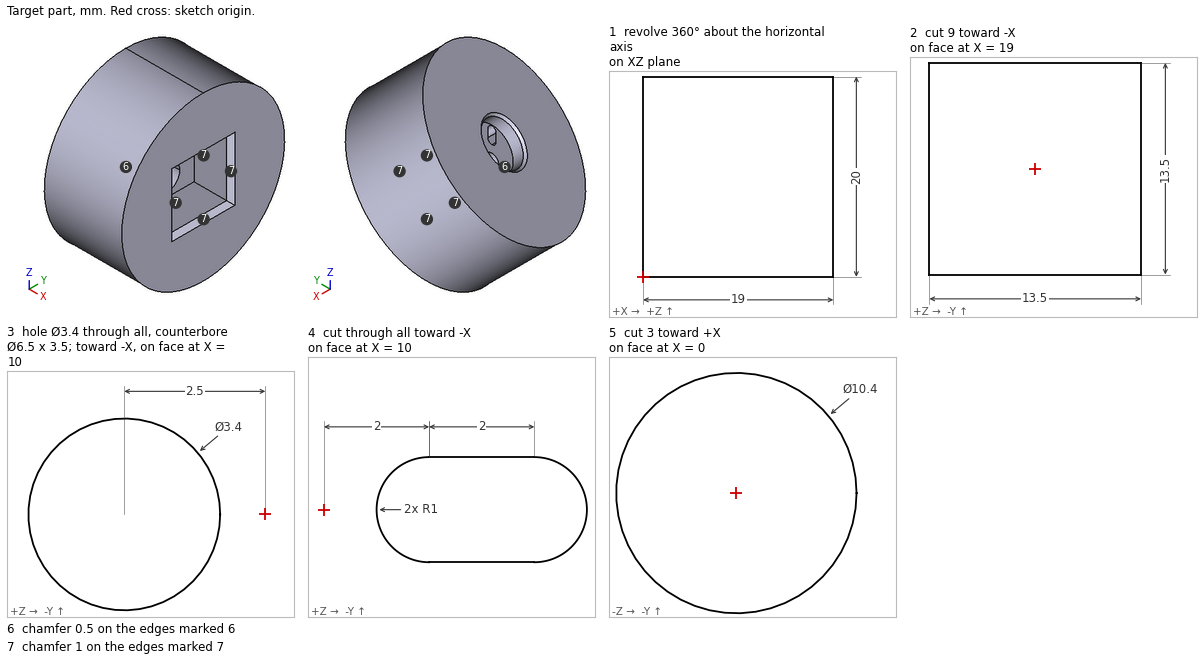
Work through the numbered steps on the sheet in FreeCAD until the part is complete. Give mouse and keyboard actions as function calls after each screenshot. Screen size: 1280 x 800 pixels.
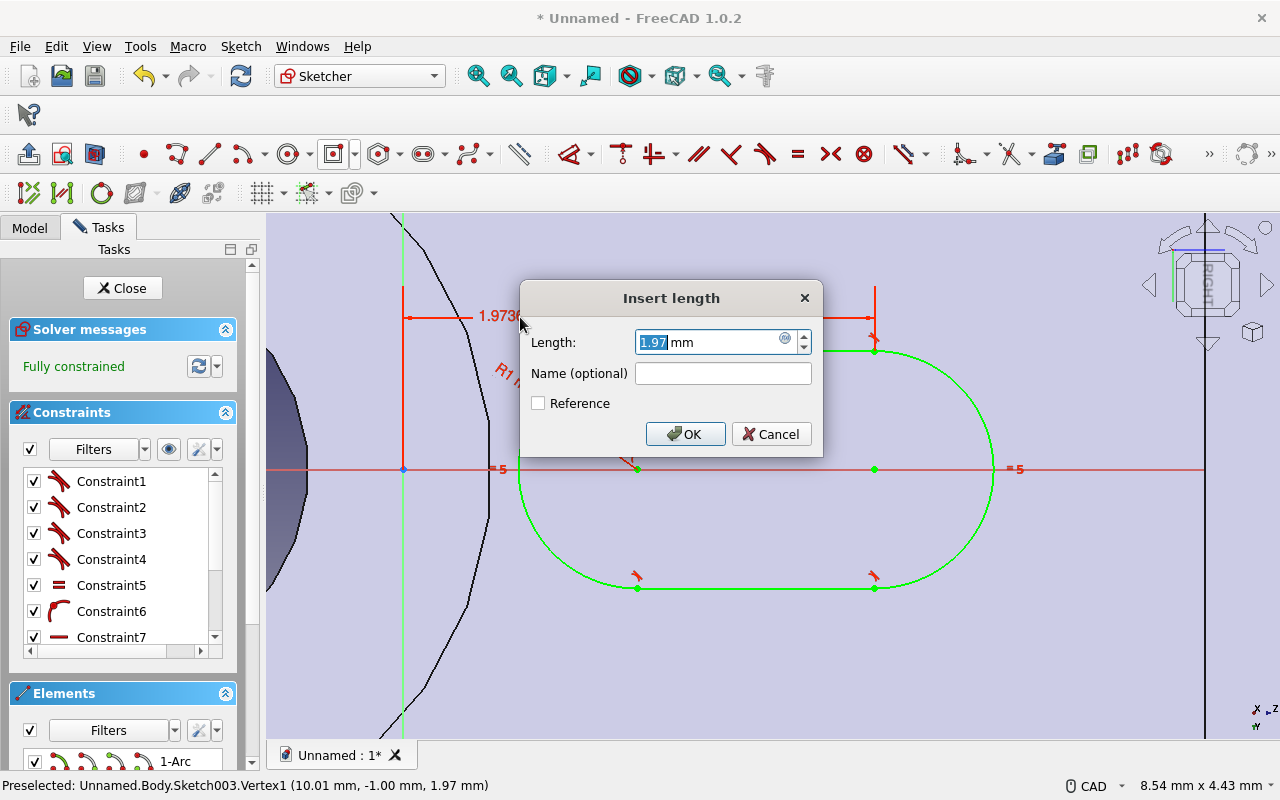
text(2)
key(Return)
key(Escape)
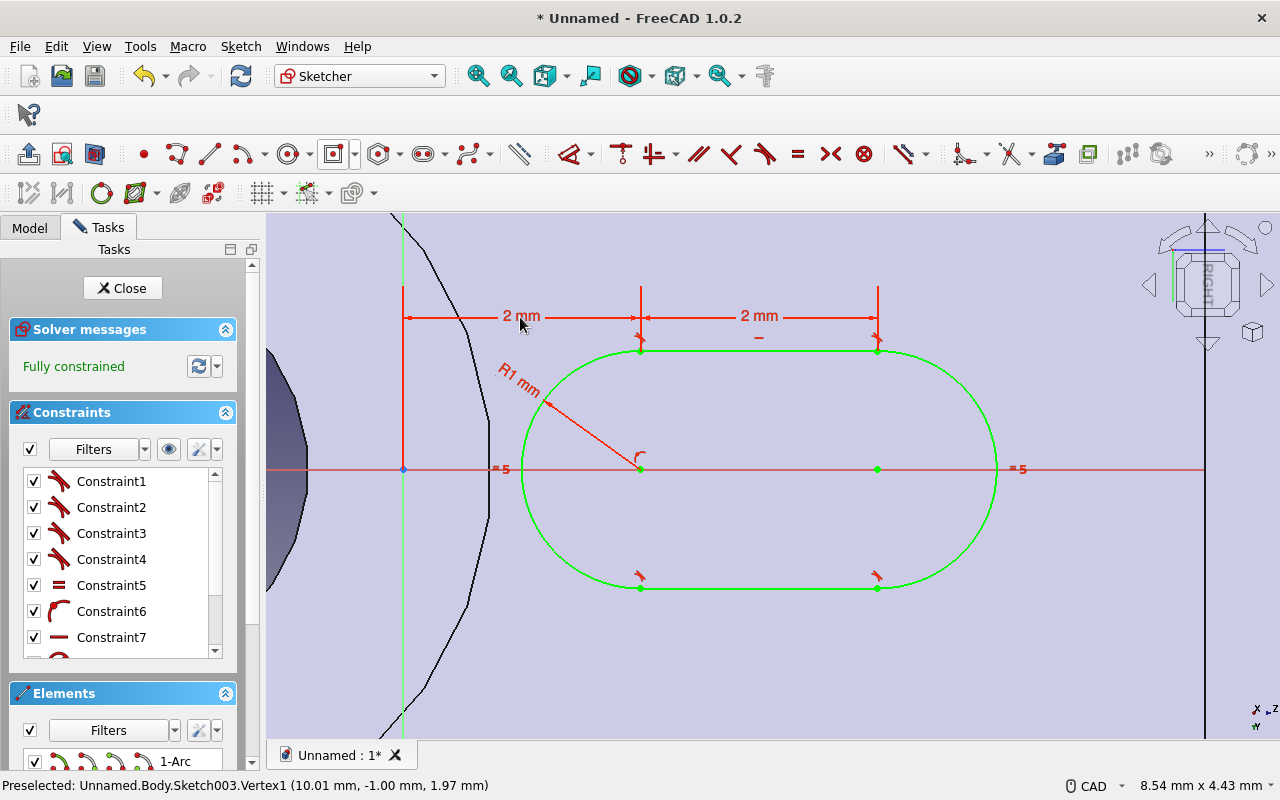
click(123, 288)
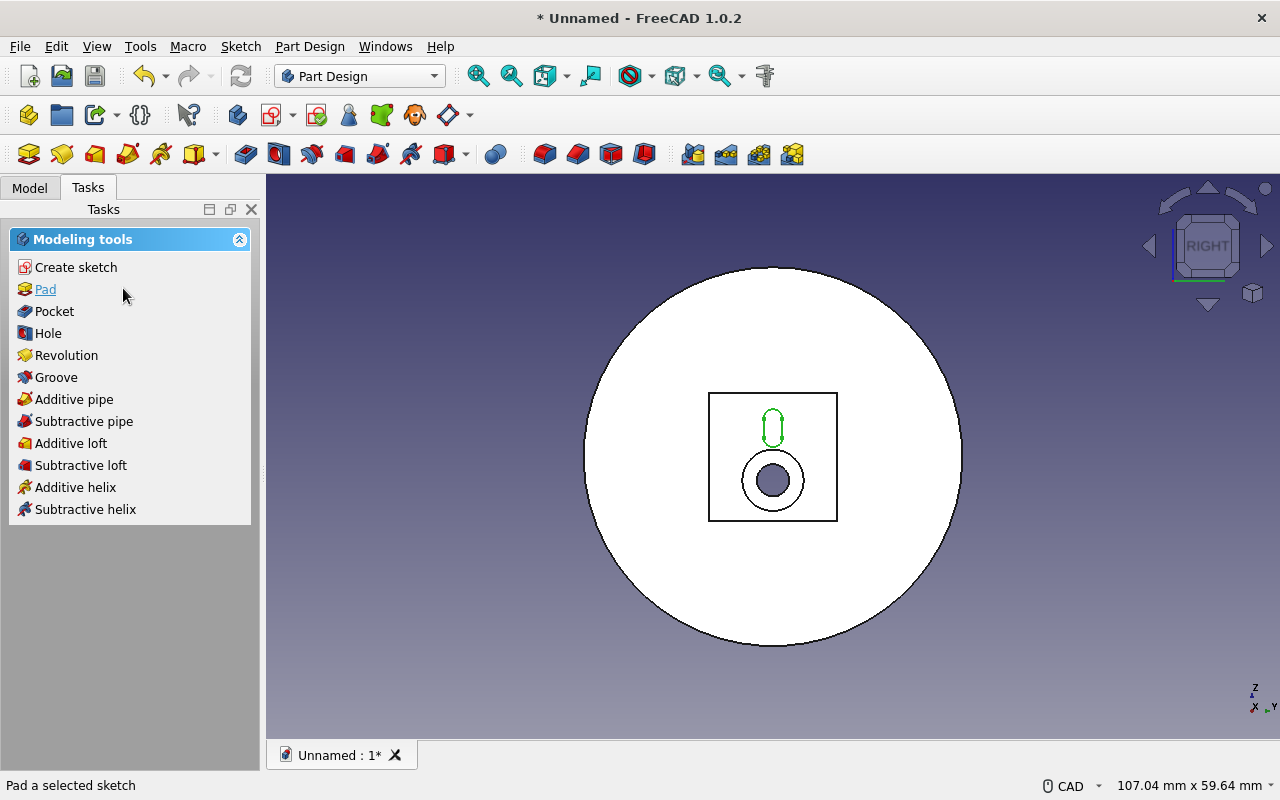
click(246, 154)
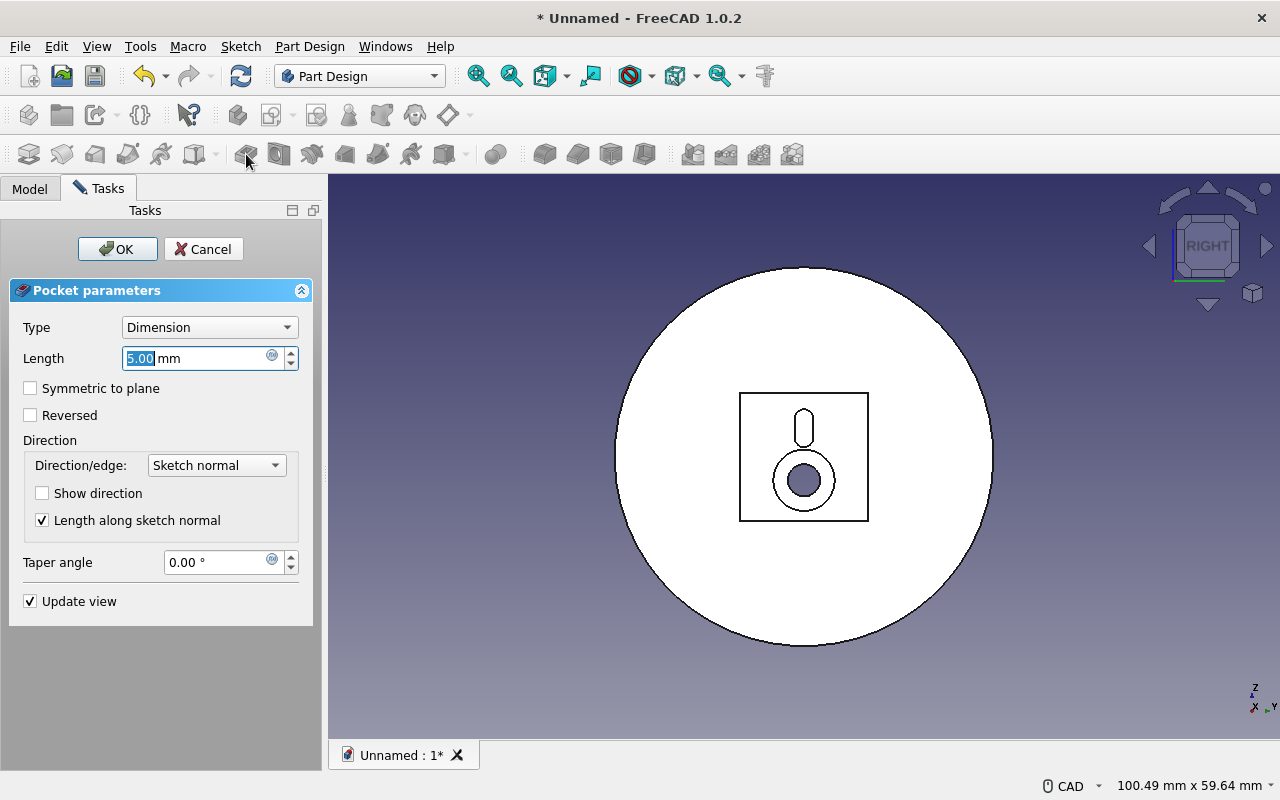
click(210, 328)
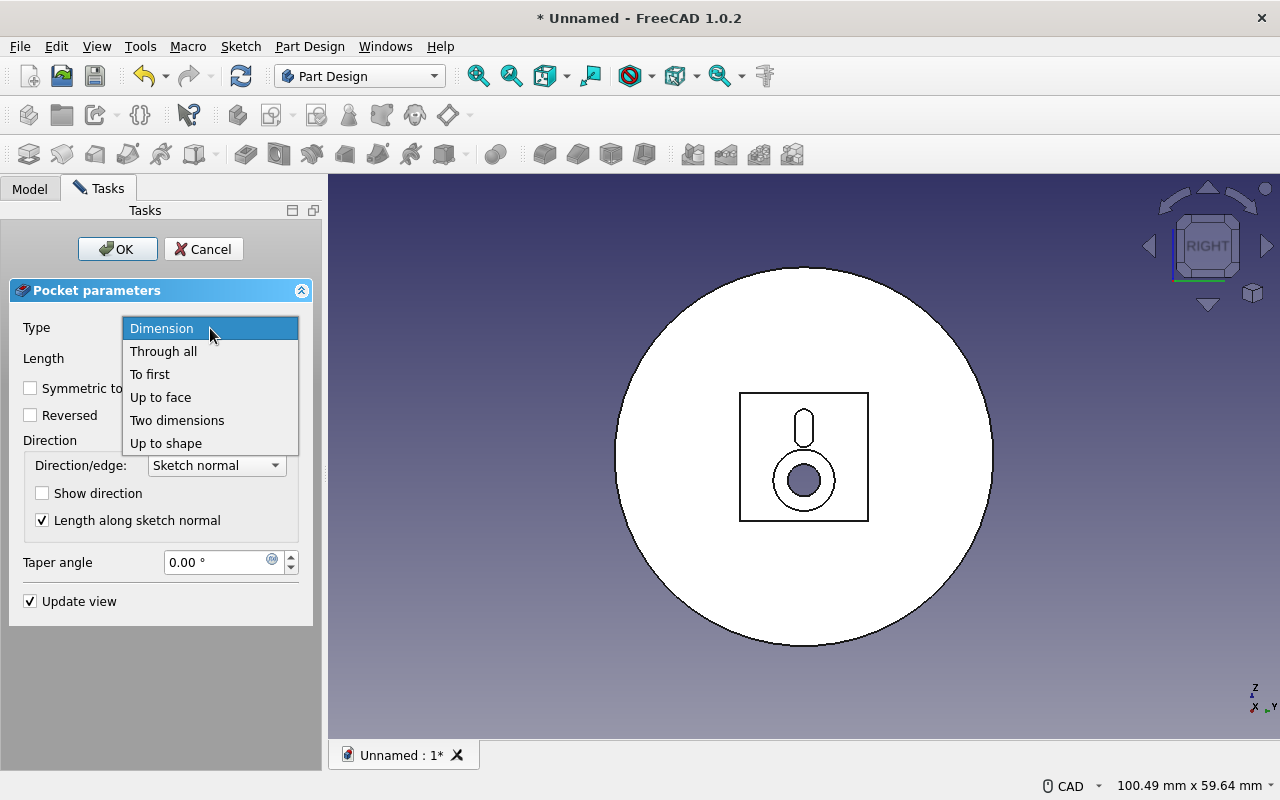
click(208, 352)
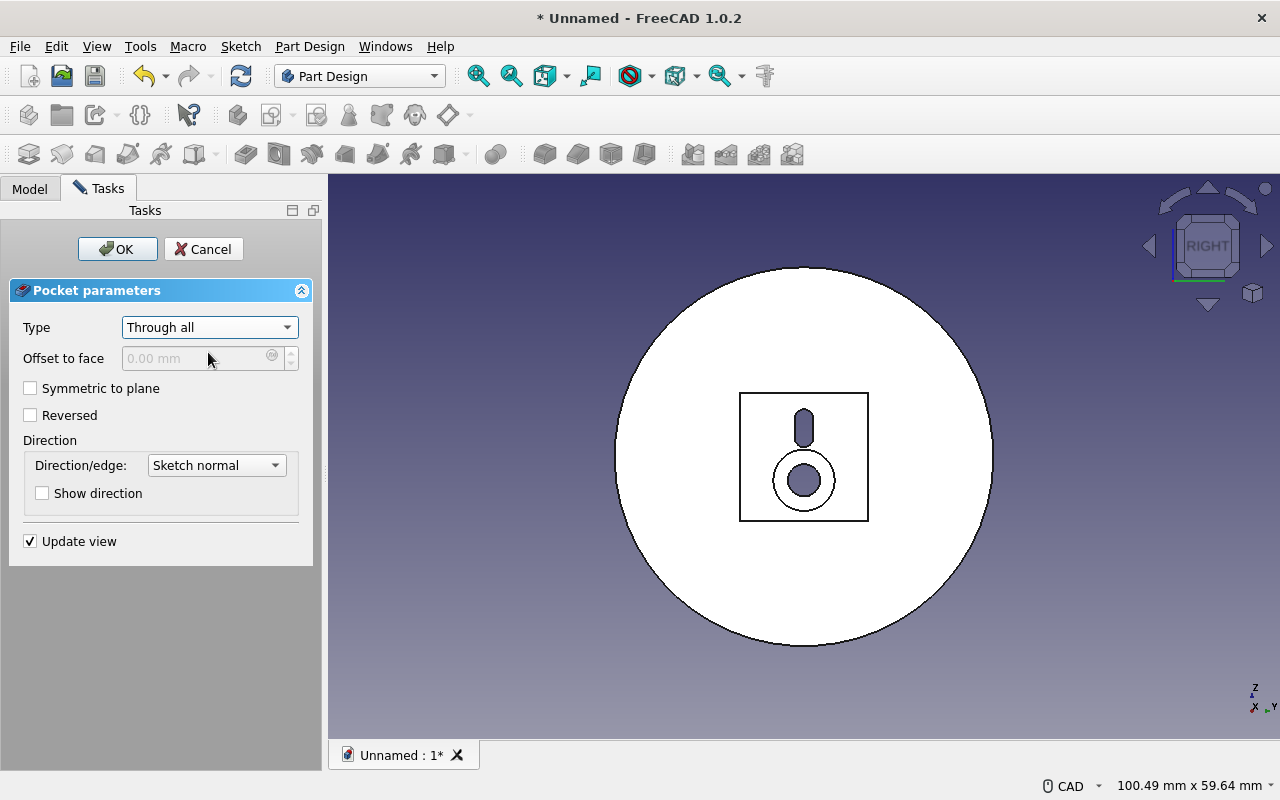
click(118, 249)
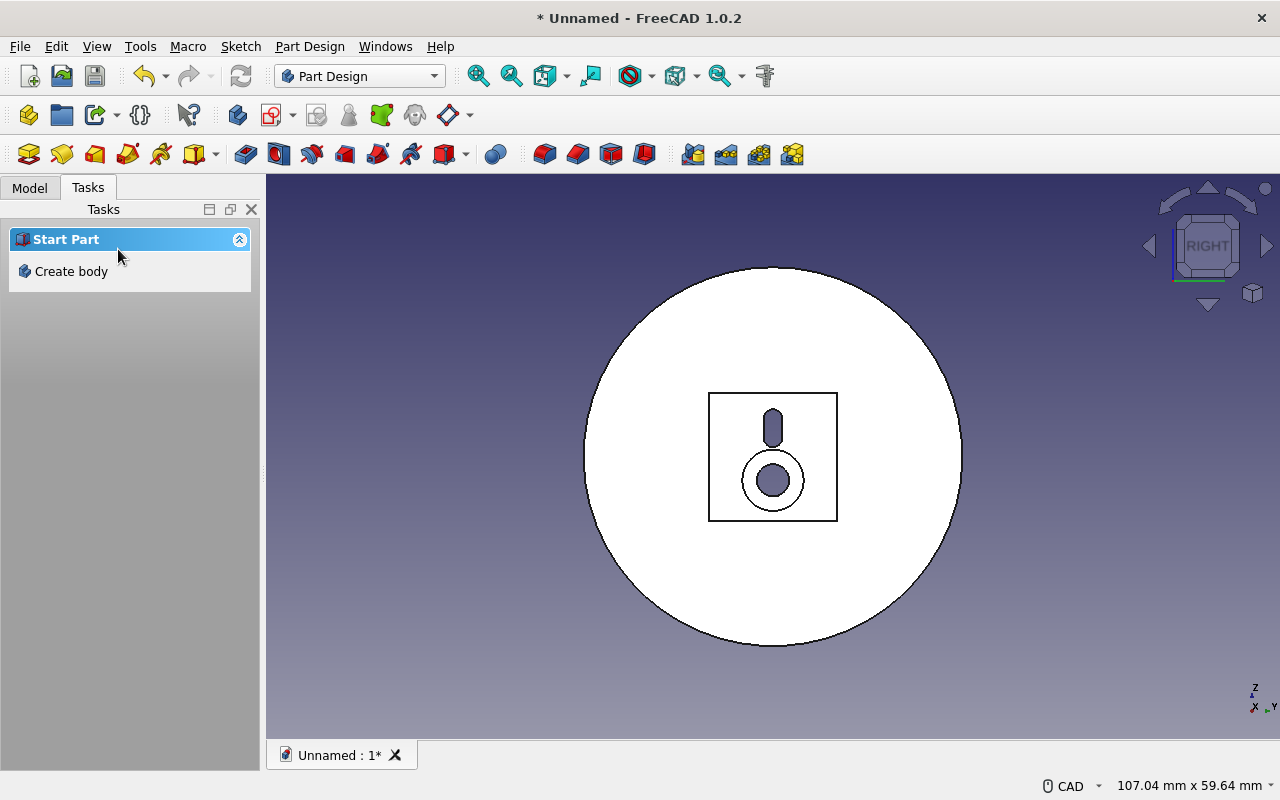
key(6)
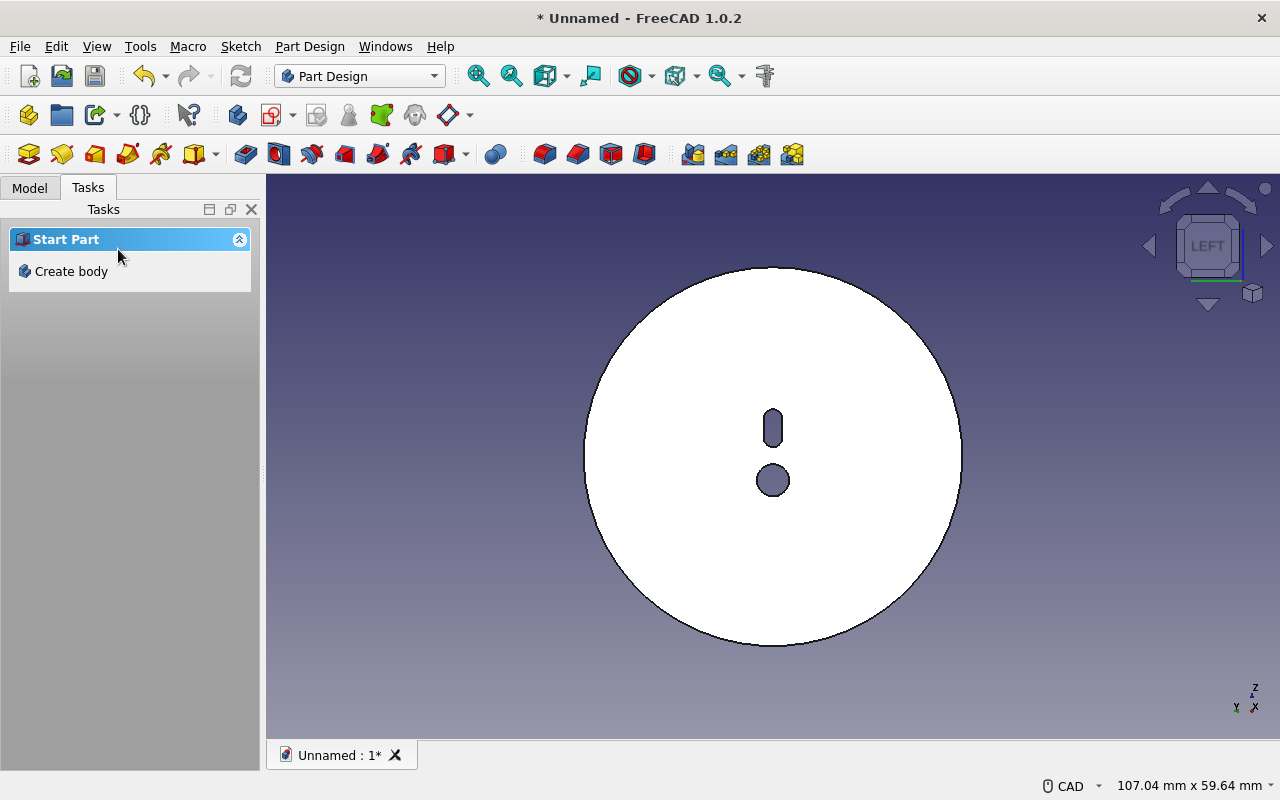
click(881, 456)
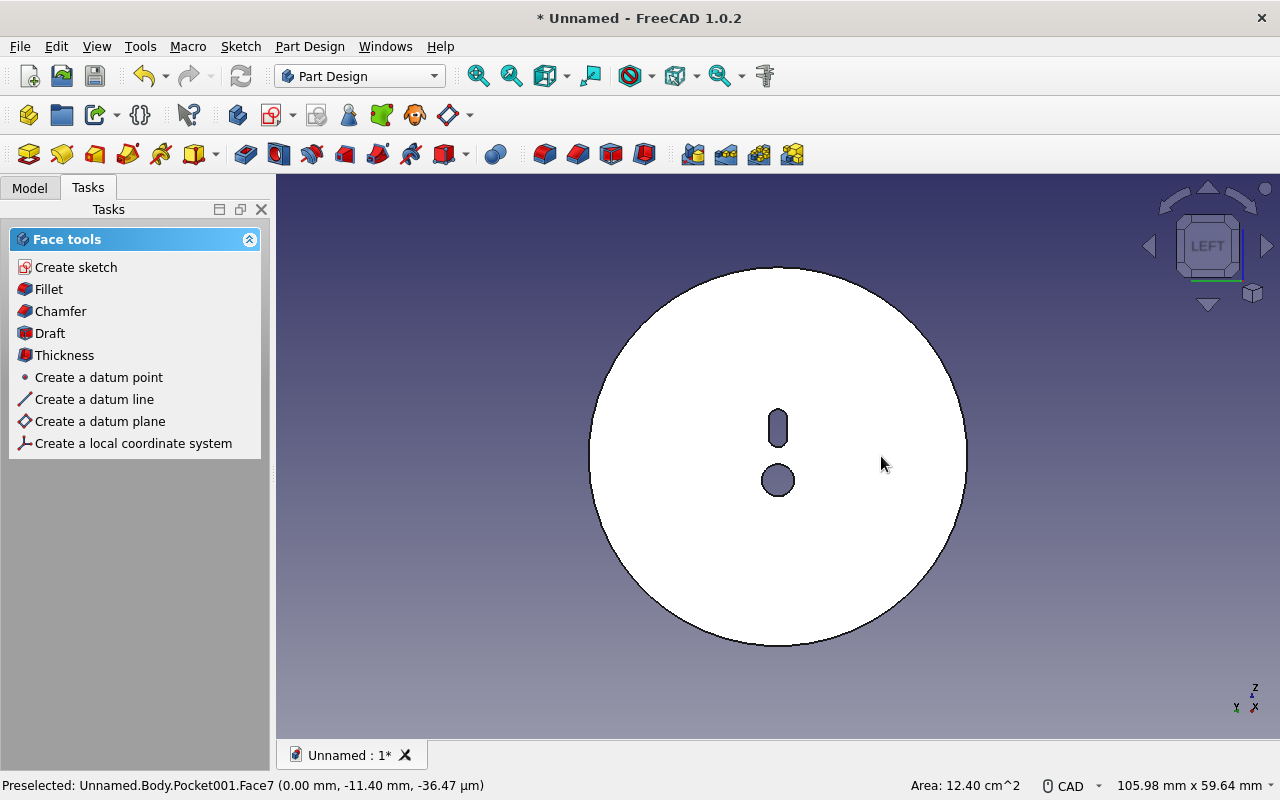
click(270, 116)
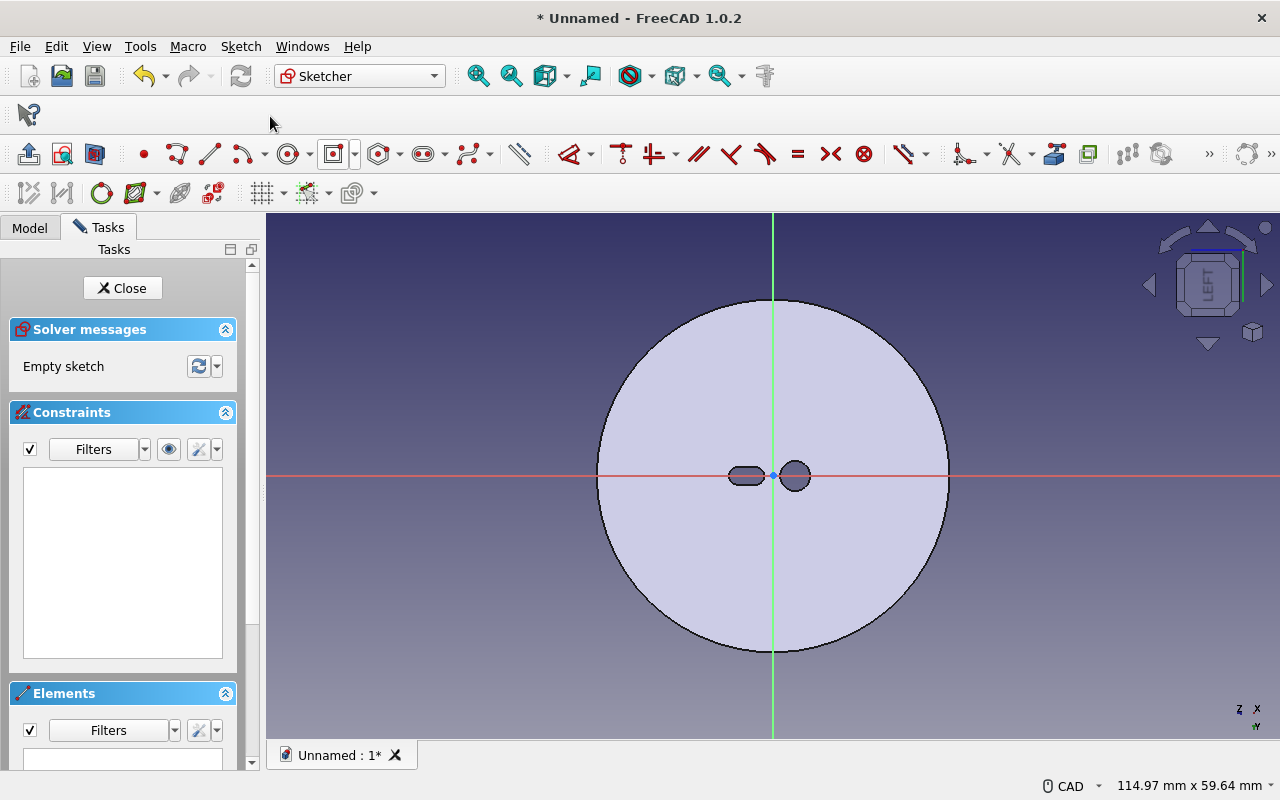
scroll(803, 476, up, 6)